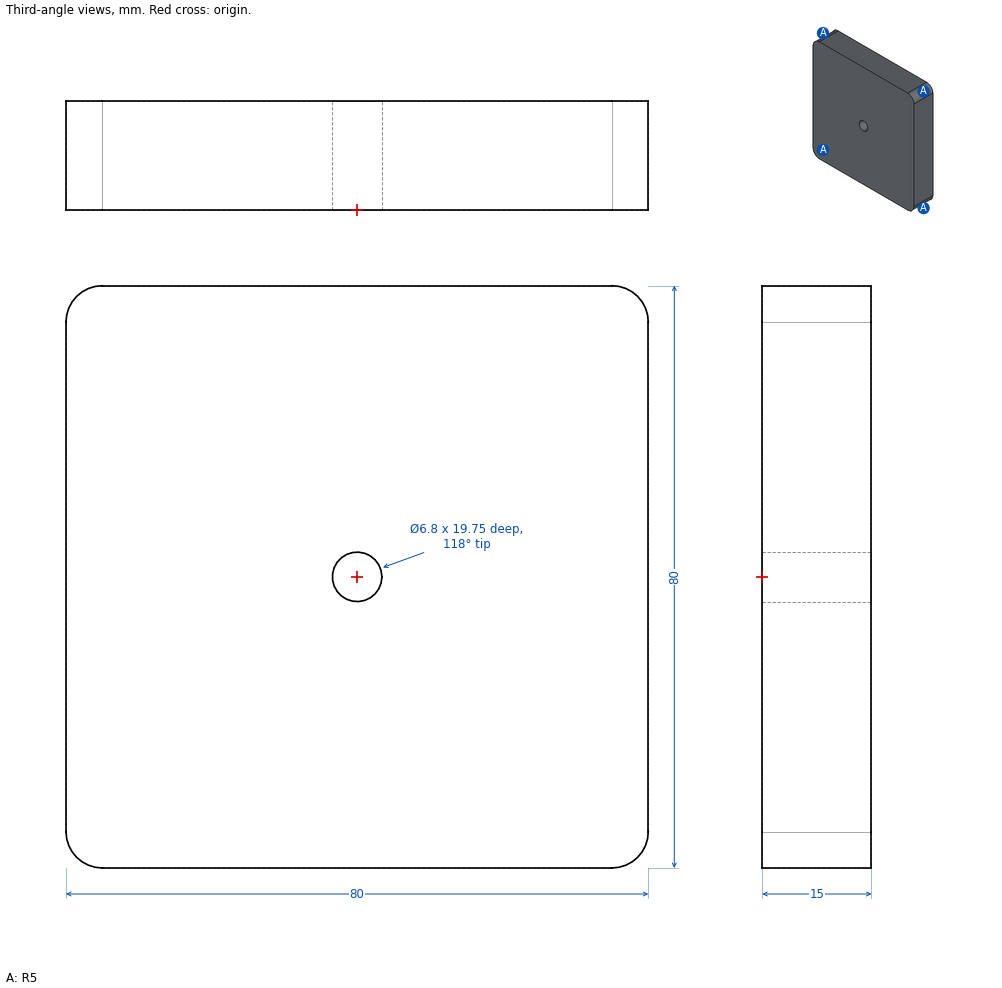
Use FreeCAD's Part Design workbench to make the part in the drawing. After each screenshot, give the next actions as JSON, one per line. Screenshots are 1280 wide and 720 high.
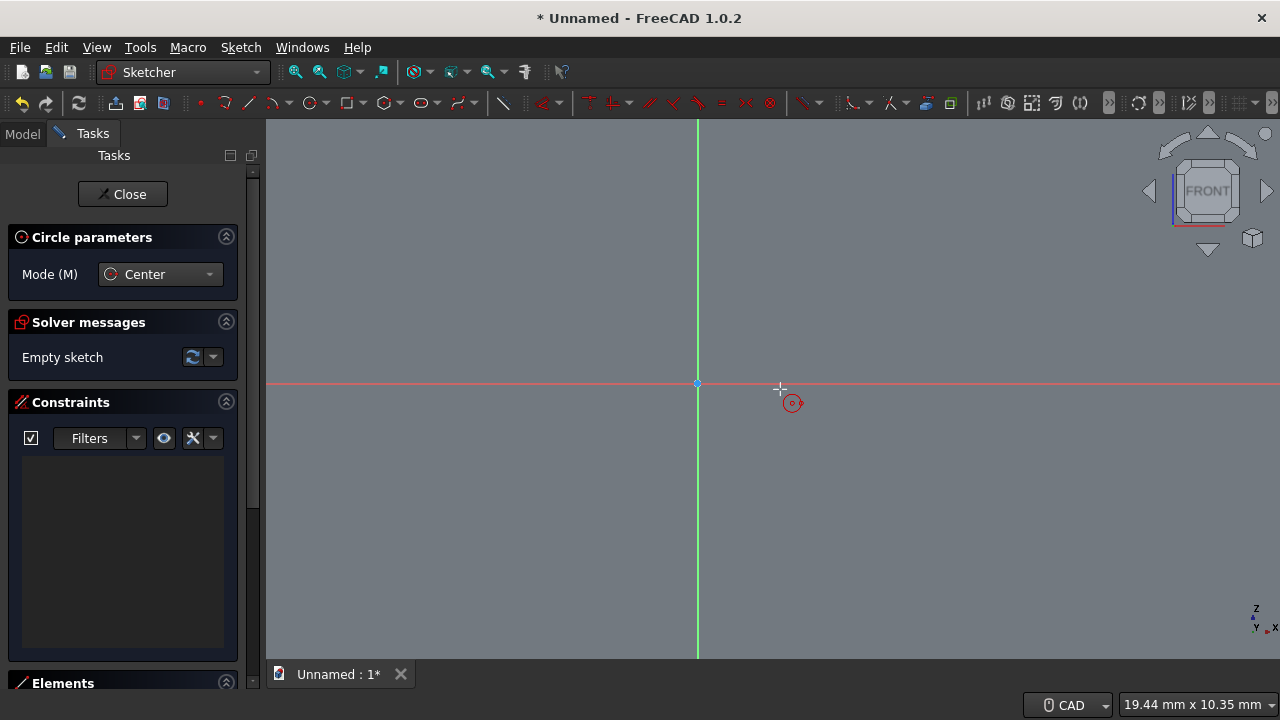
{"action": "left_click", "coordinate": [698, 384]}
{"action": "mouse_move", "coordinate": [823, 259]}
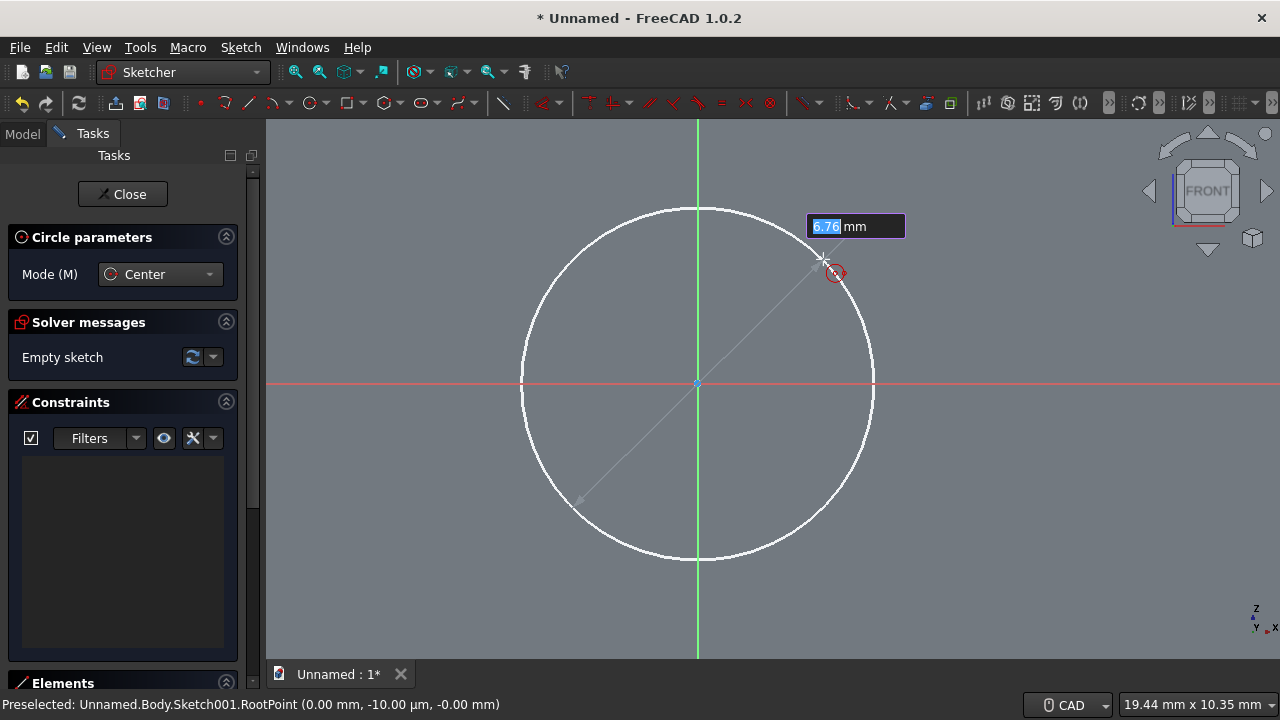
{"action": "type", "text": "6.8"}
{"action": "key", "text": "Return"}
{"action": "key", "text": "Escape"}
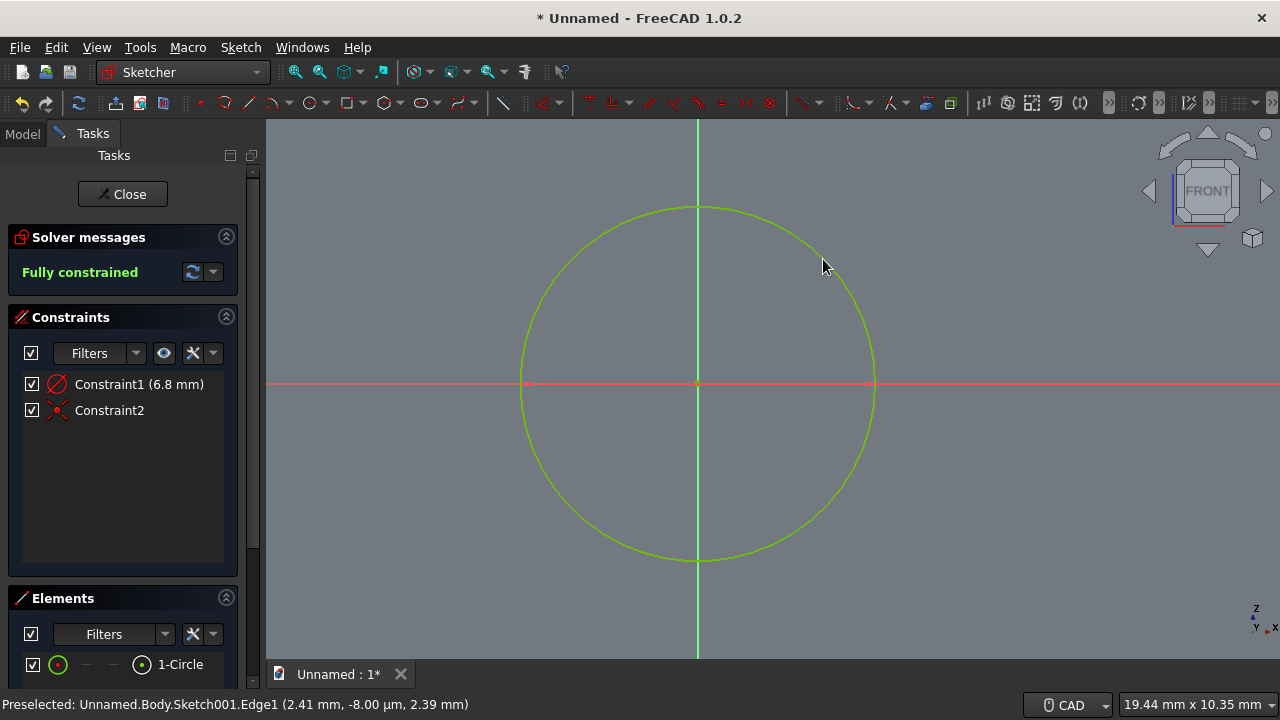
{"action": "left_click", "coordinate": [123, 194]}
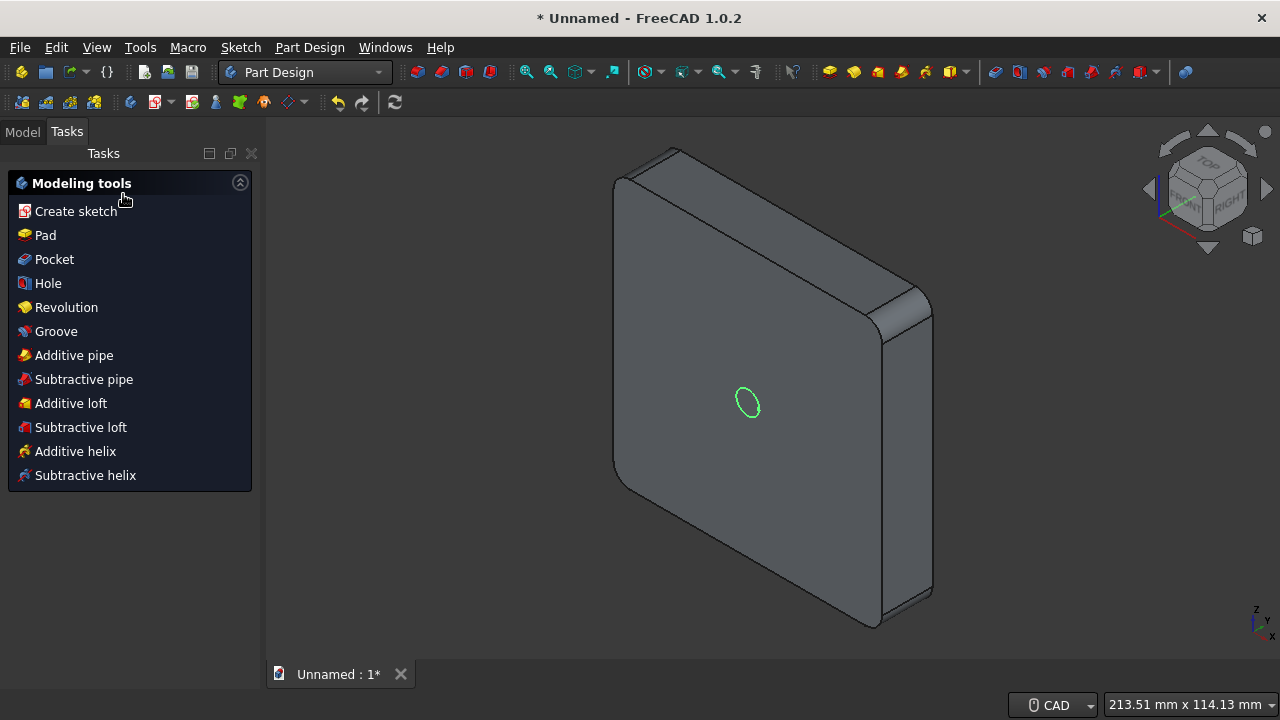
{"action": "left_click", "coordinate": [1020, 72]}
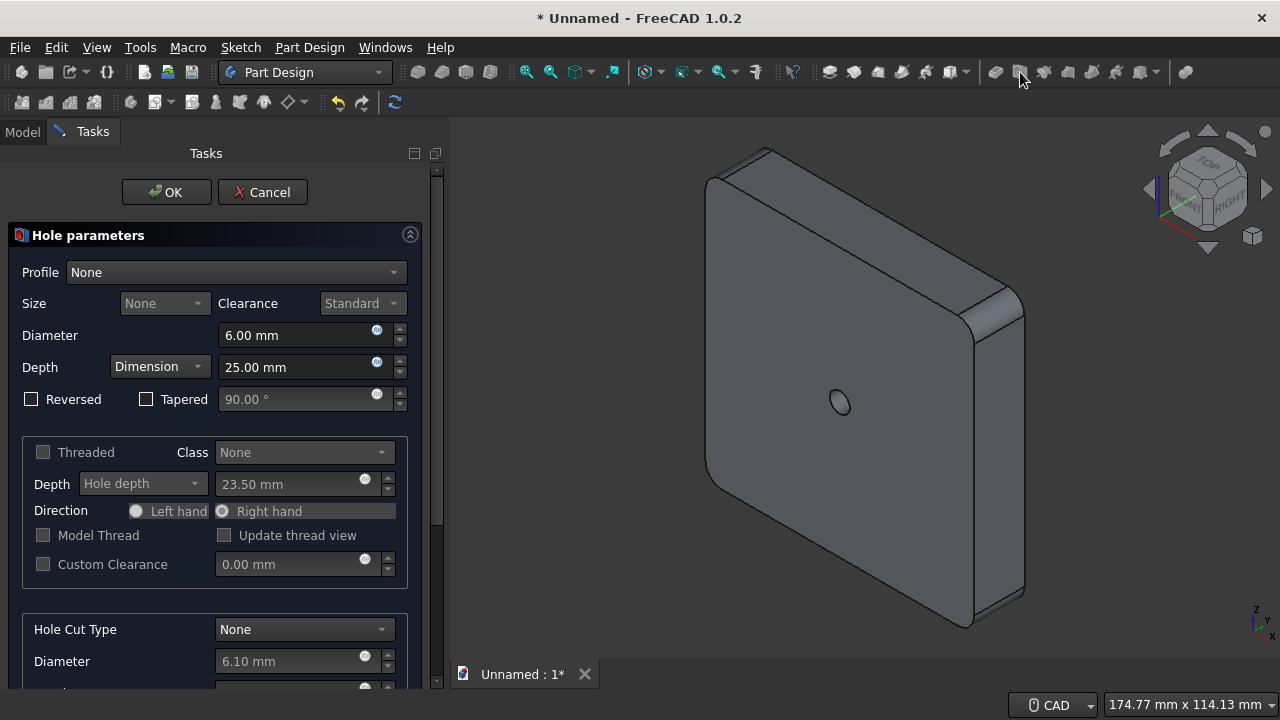
{"action": "triple_click", "coordinate": [305, 335]}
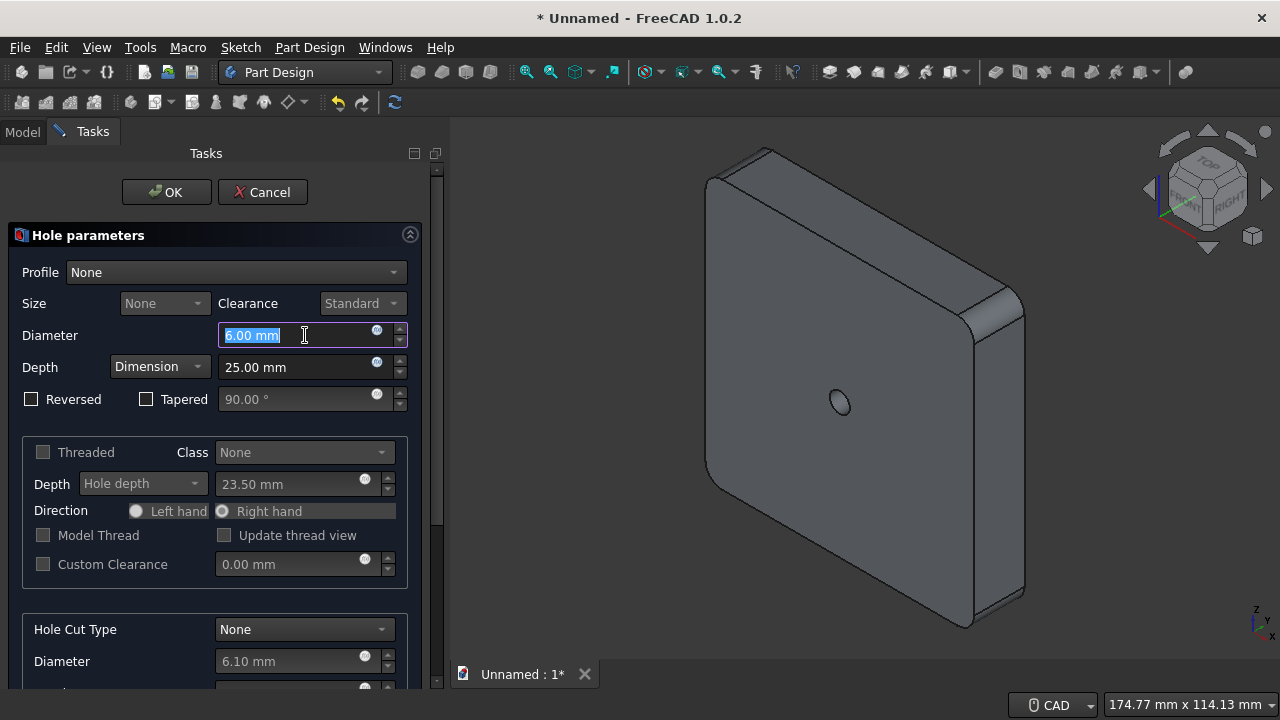
{"action": "type", "text": "6.8"}
{"action": "key", "text": "Tab"}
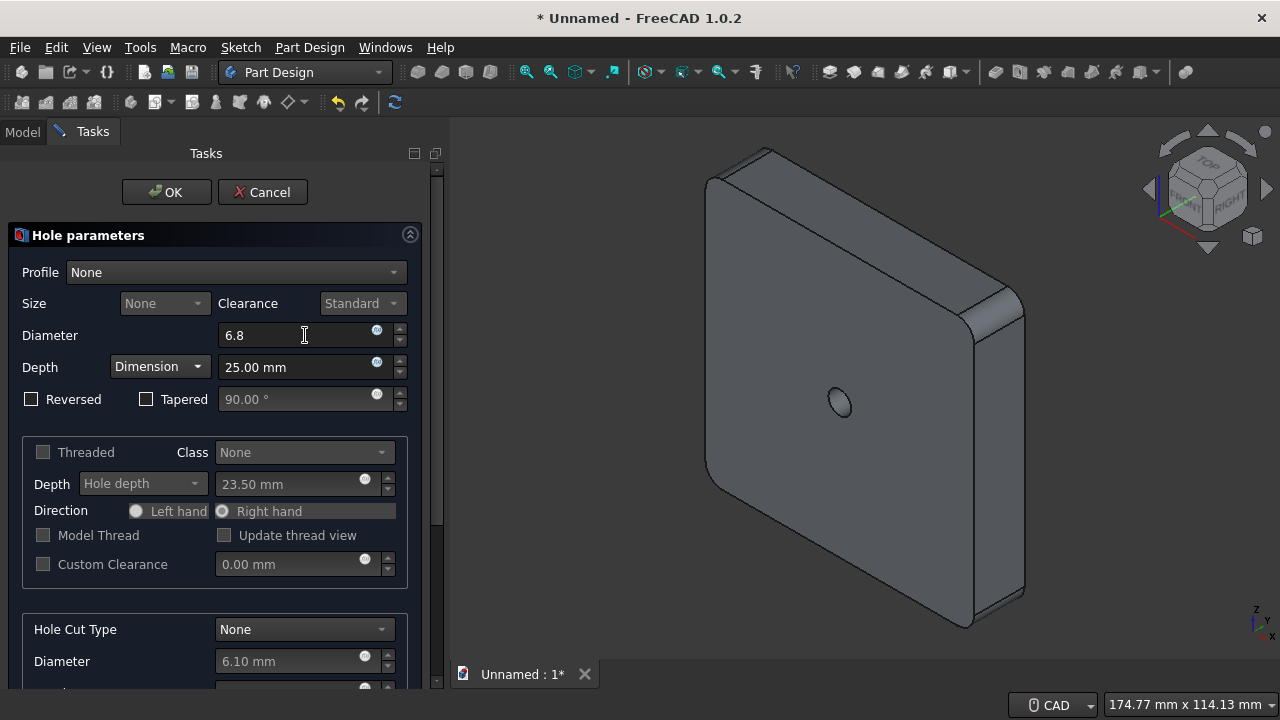
{"action": "triple_click", "coordinate": [305, 367]}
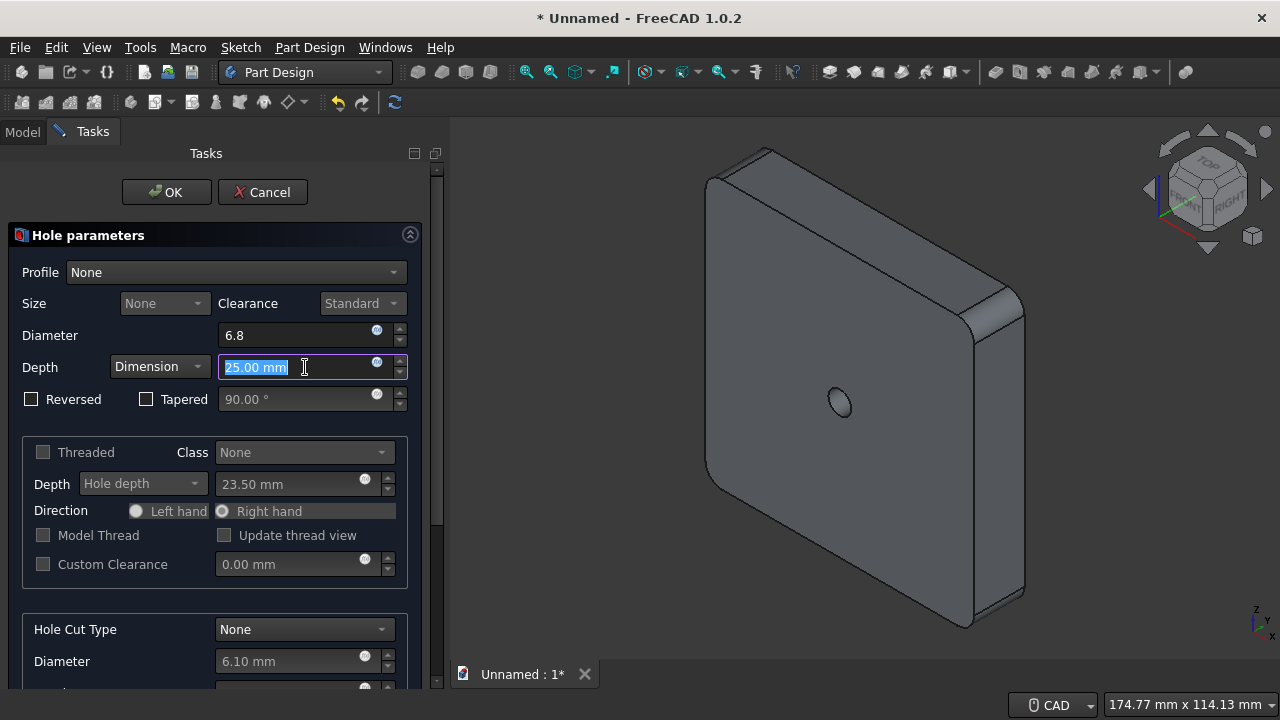
{"action": "type", "text": "19.75"}
{"action": "key", "text": "Tab"}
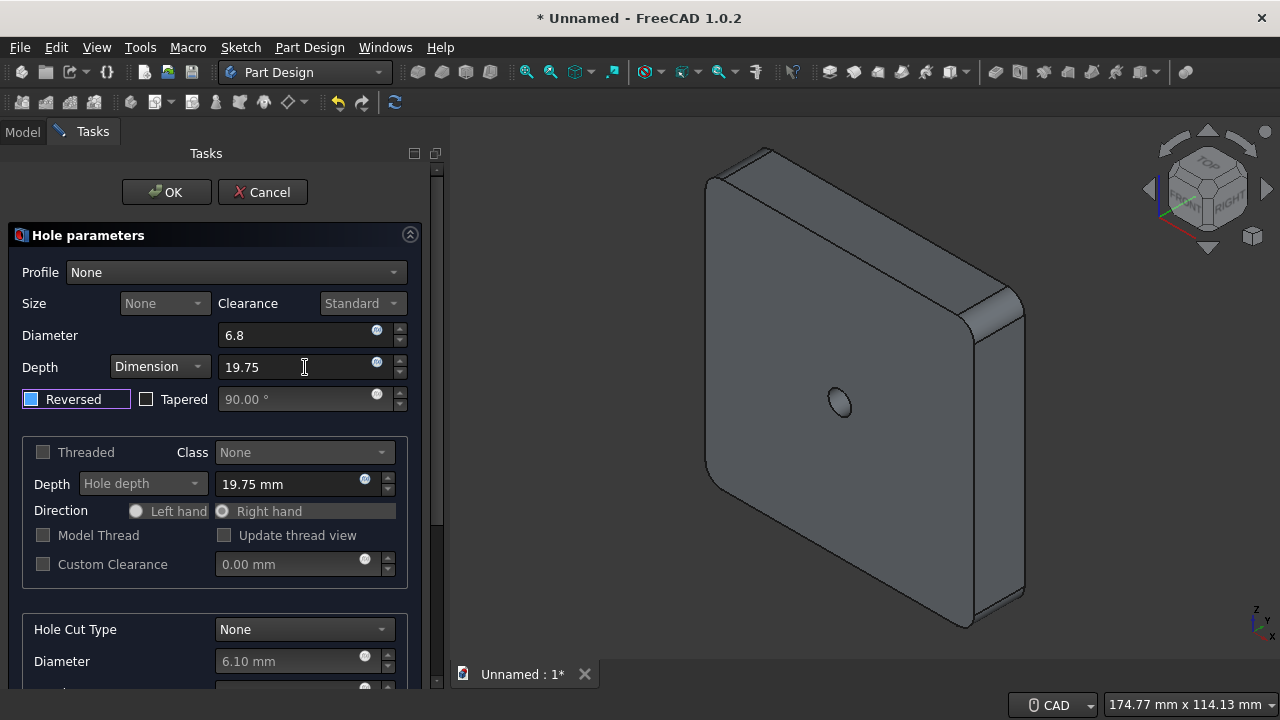
{"action": "left_click", "coordinate": [167, 192]}